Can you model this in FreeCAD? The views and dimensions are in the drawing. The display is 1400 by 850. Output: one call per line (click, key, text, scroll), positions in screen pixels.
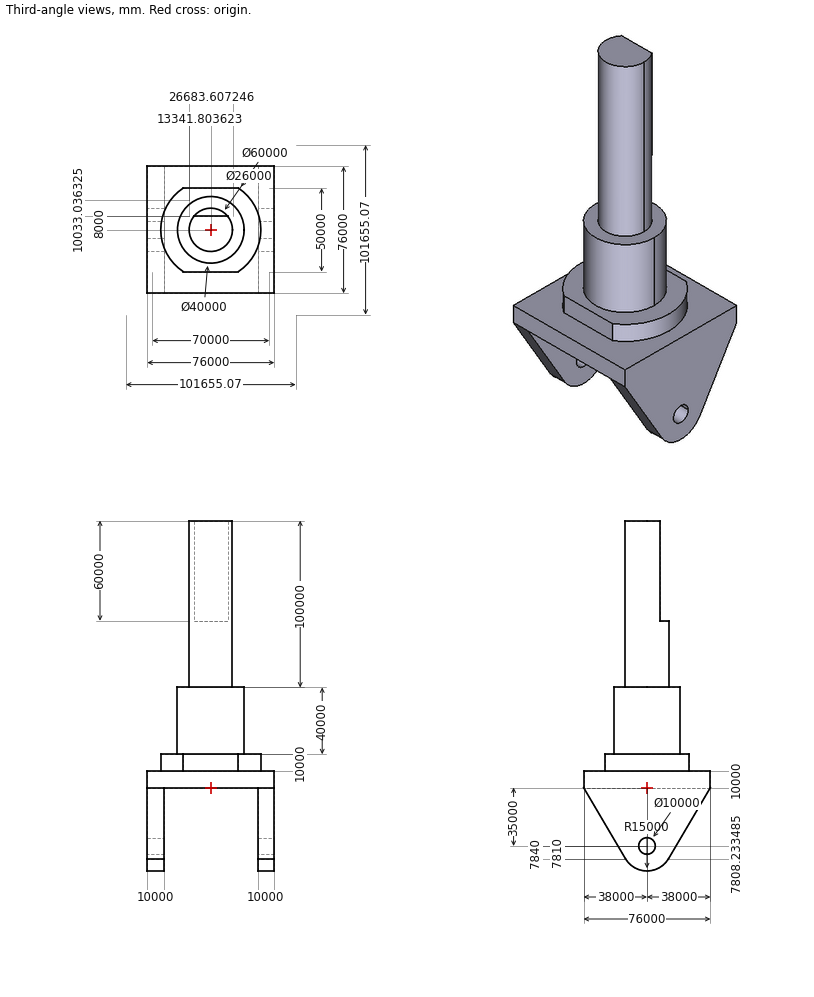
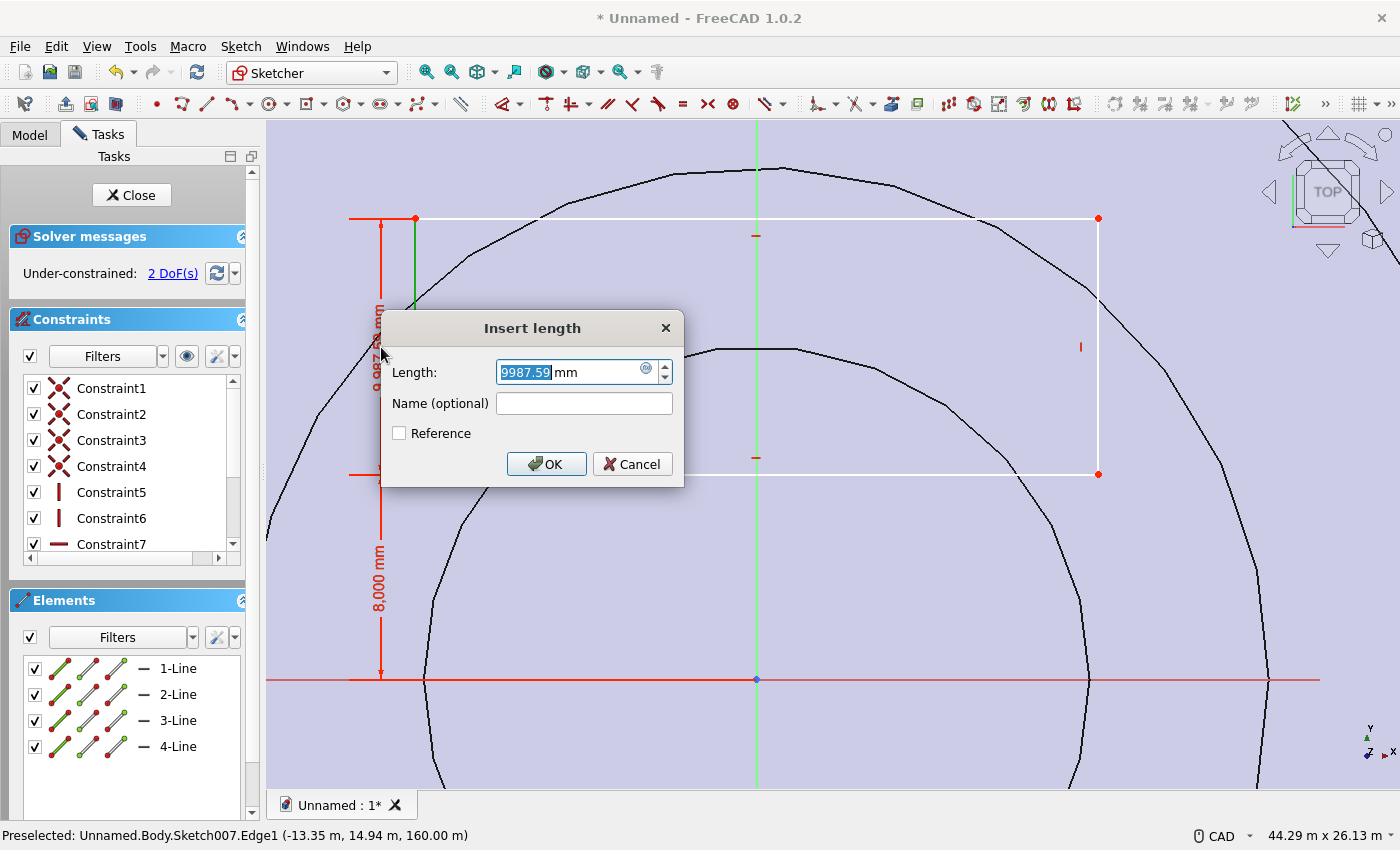
text(10033.036325)
key(Return)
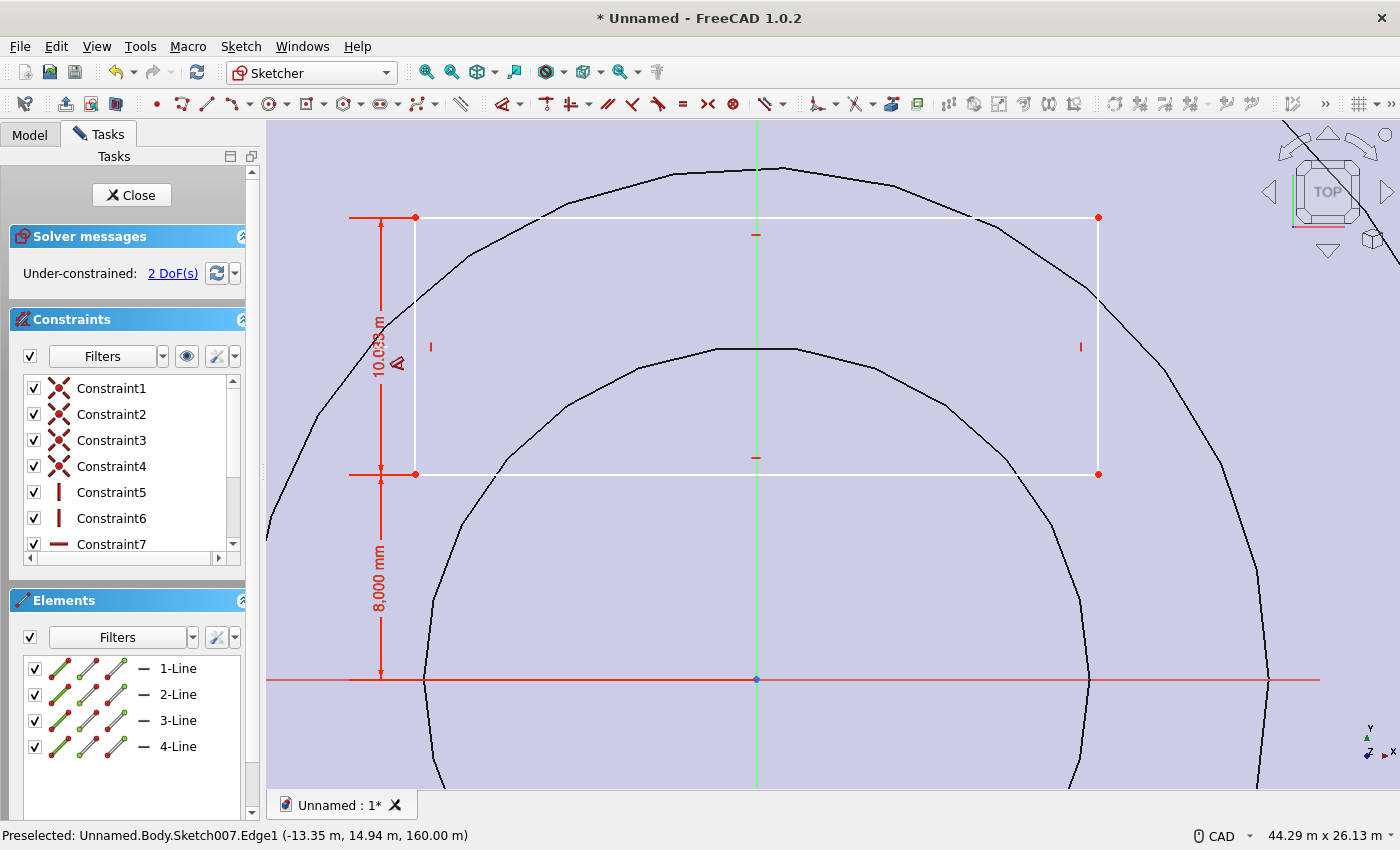
click(620, 475)
click(599, 509)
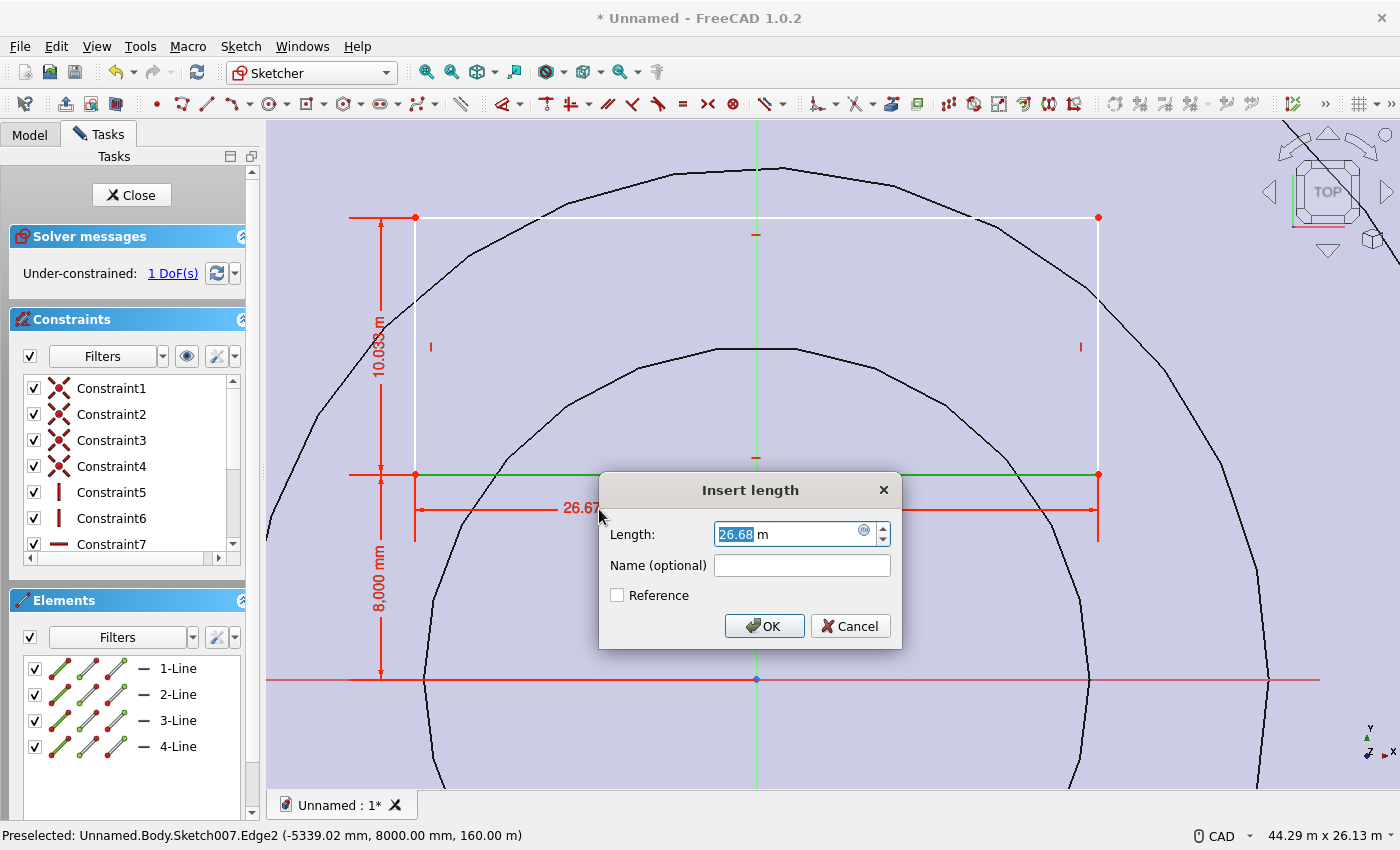
key(ctrl+a)
text(26683.607246 mm)
key(Return)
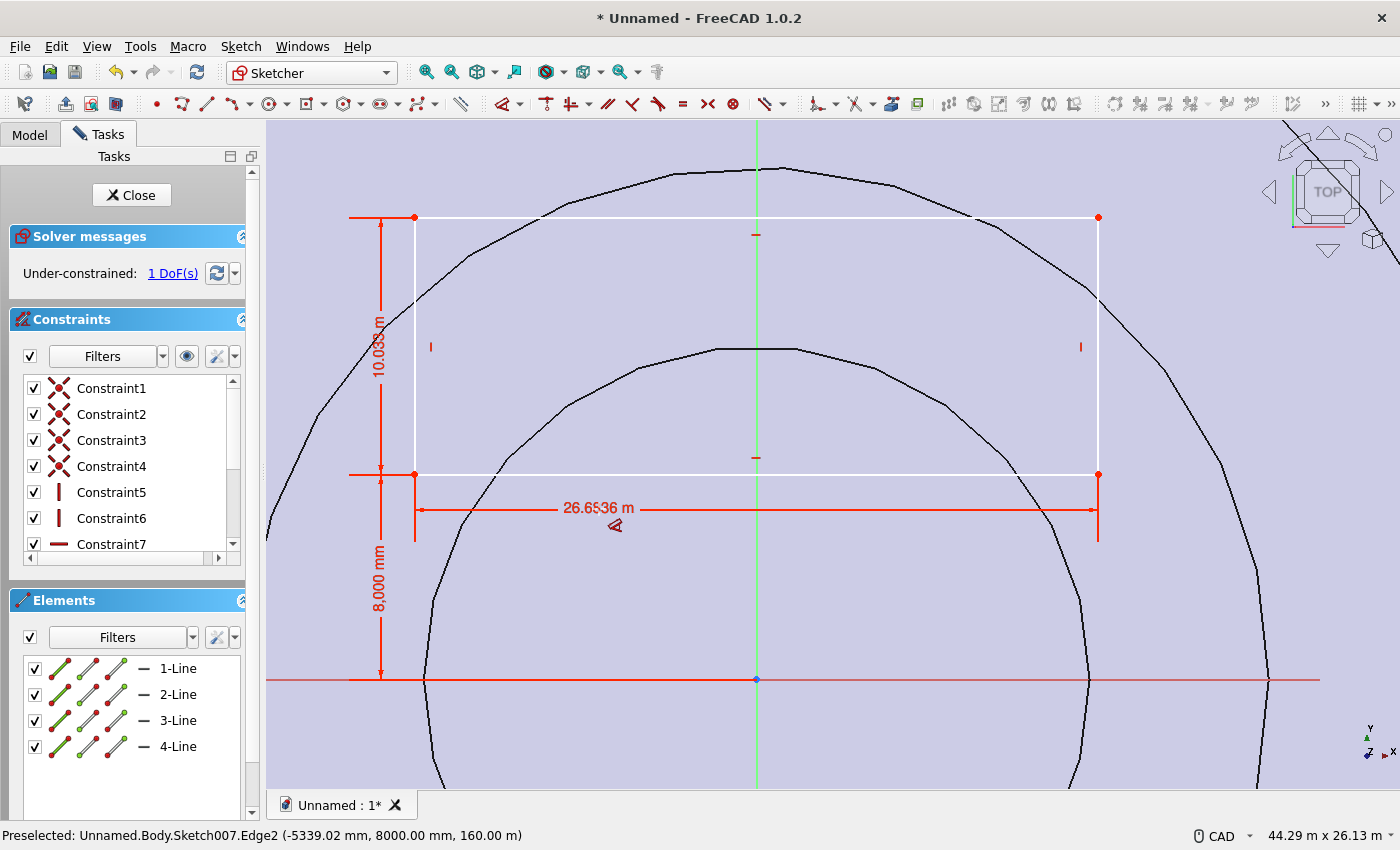
click(415, 218)
click(586, 184)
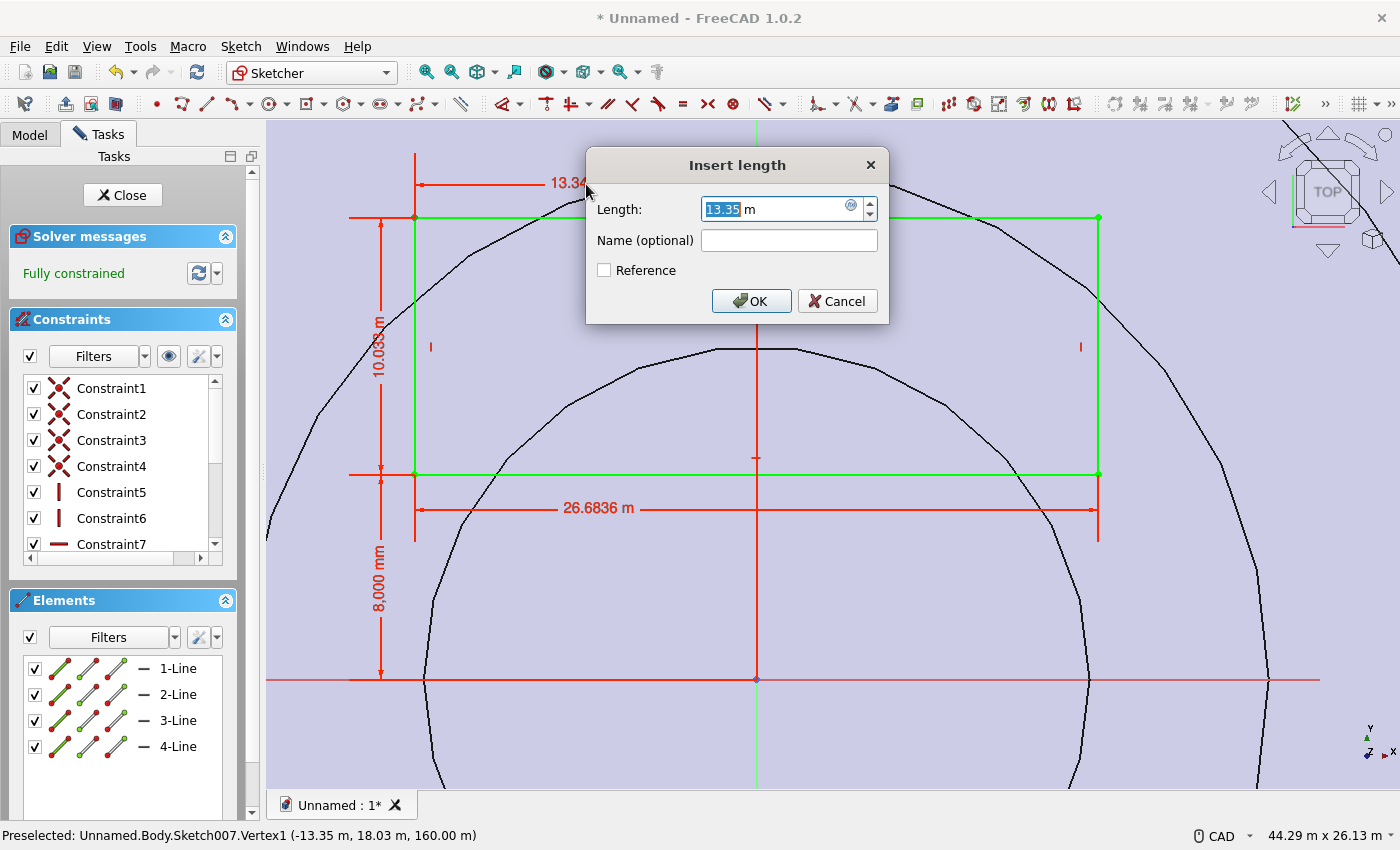
key(ctrl+a)
text(13341.803623 mm)
key(Return)
key(Escape)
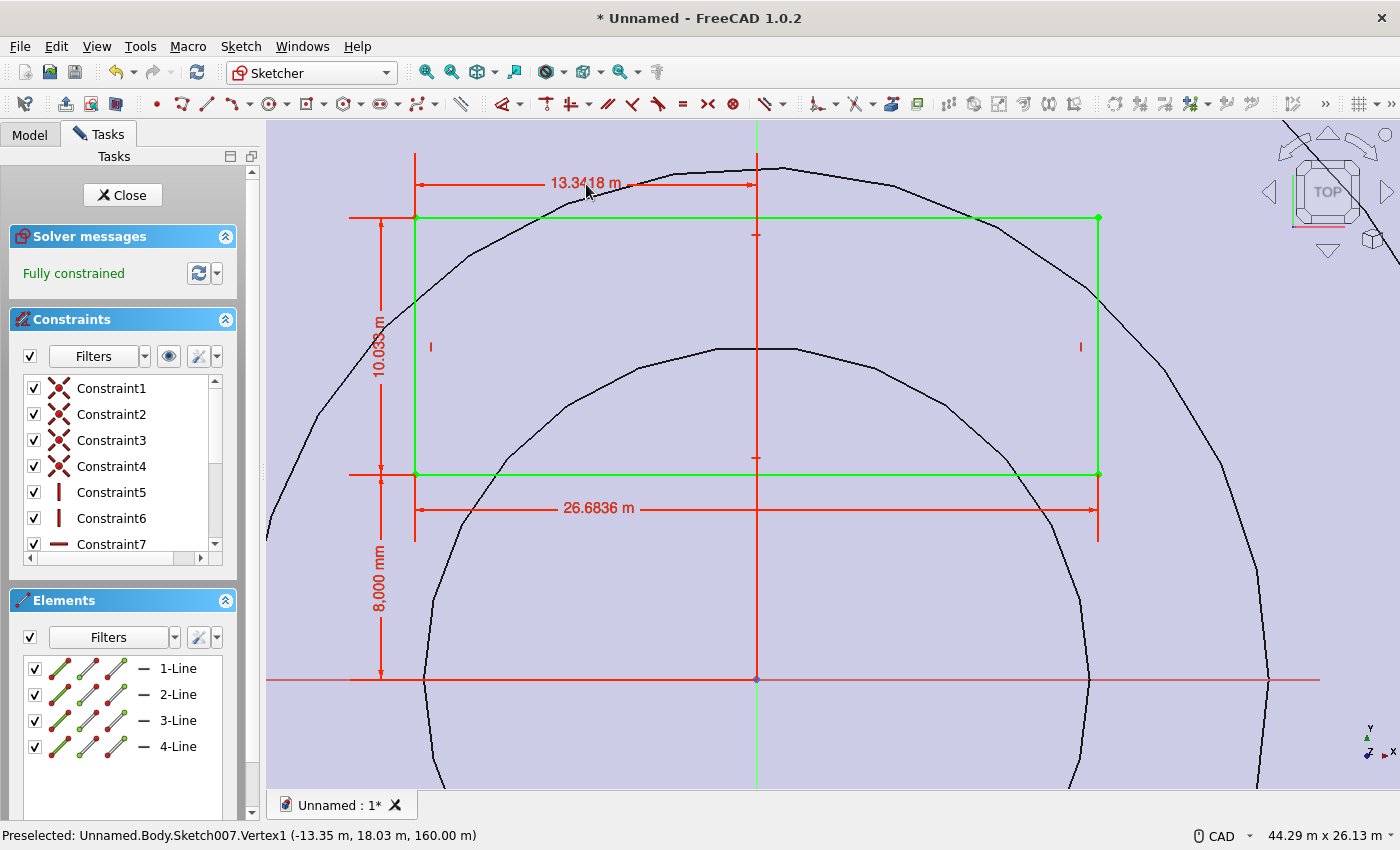
click(123, 195)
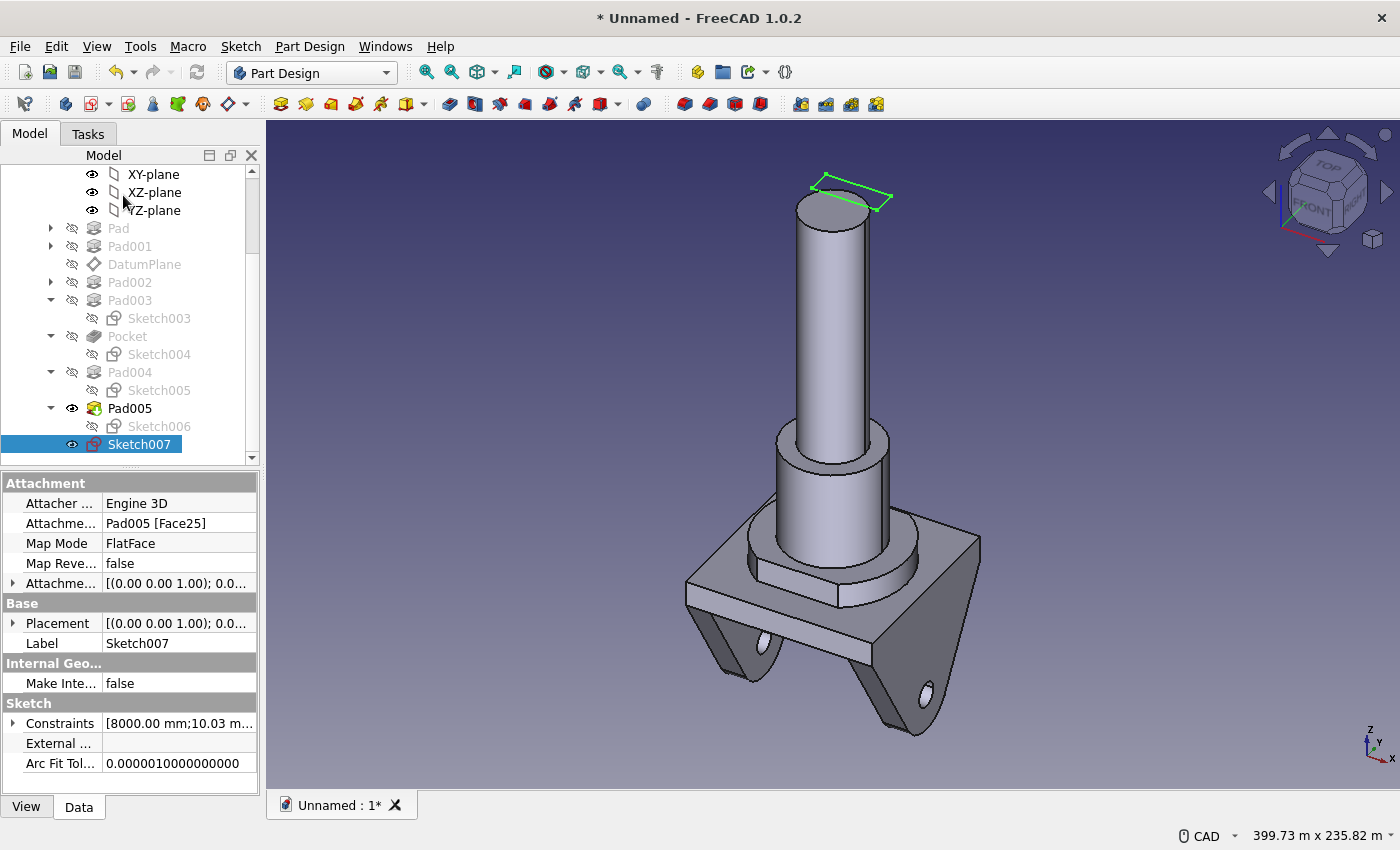
click(450, 104)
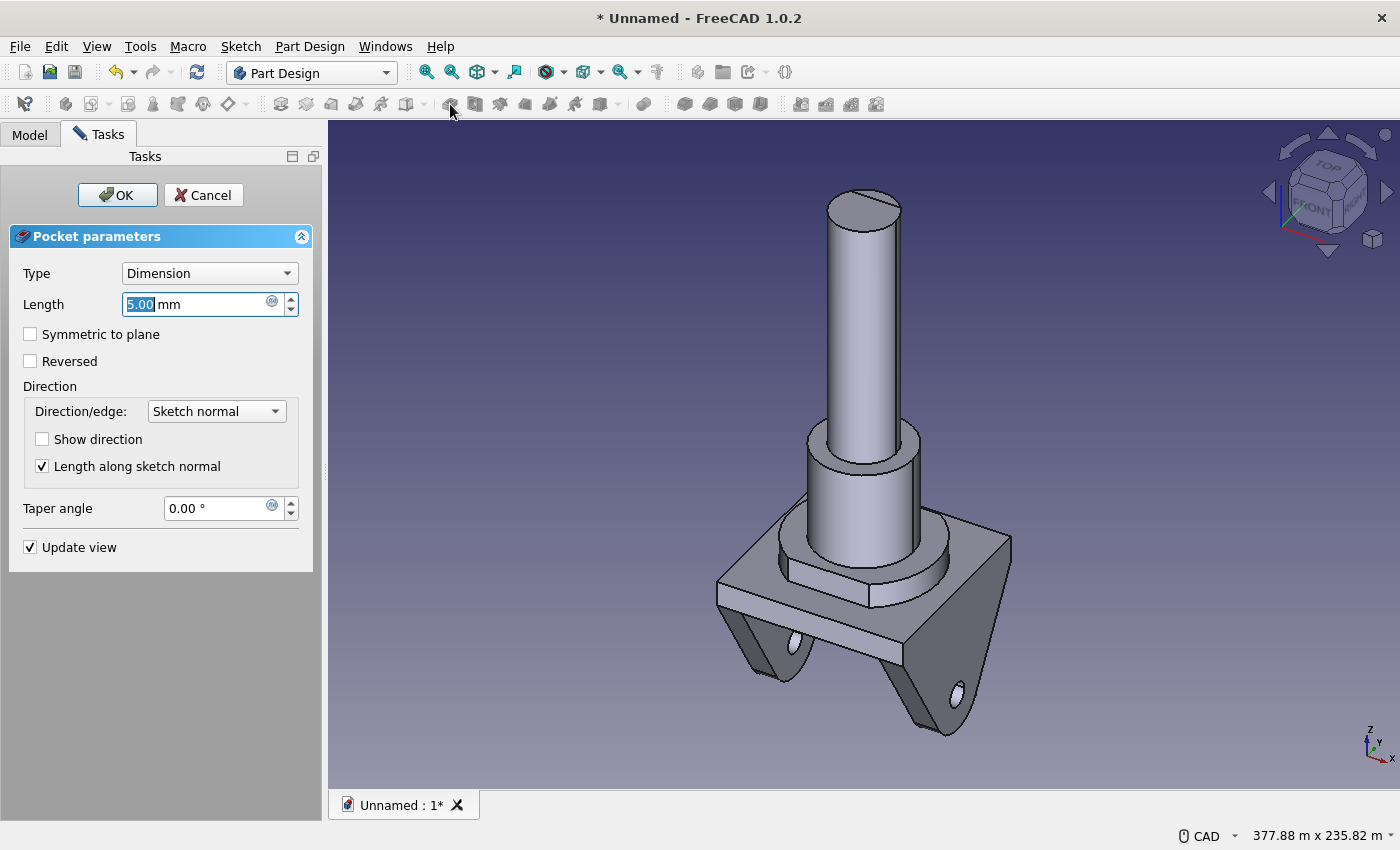
text(60000)
key(Tab)